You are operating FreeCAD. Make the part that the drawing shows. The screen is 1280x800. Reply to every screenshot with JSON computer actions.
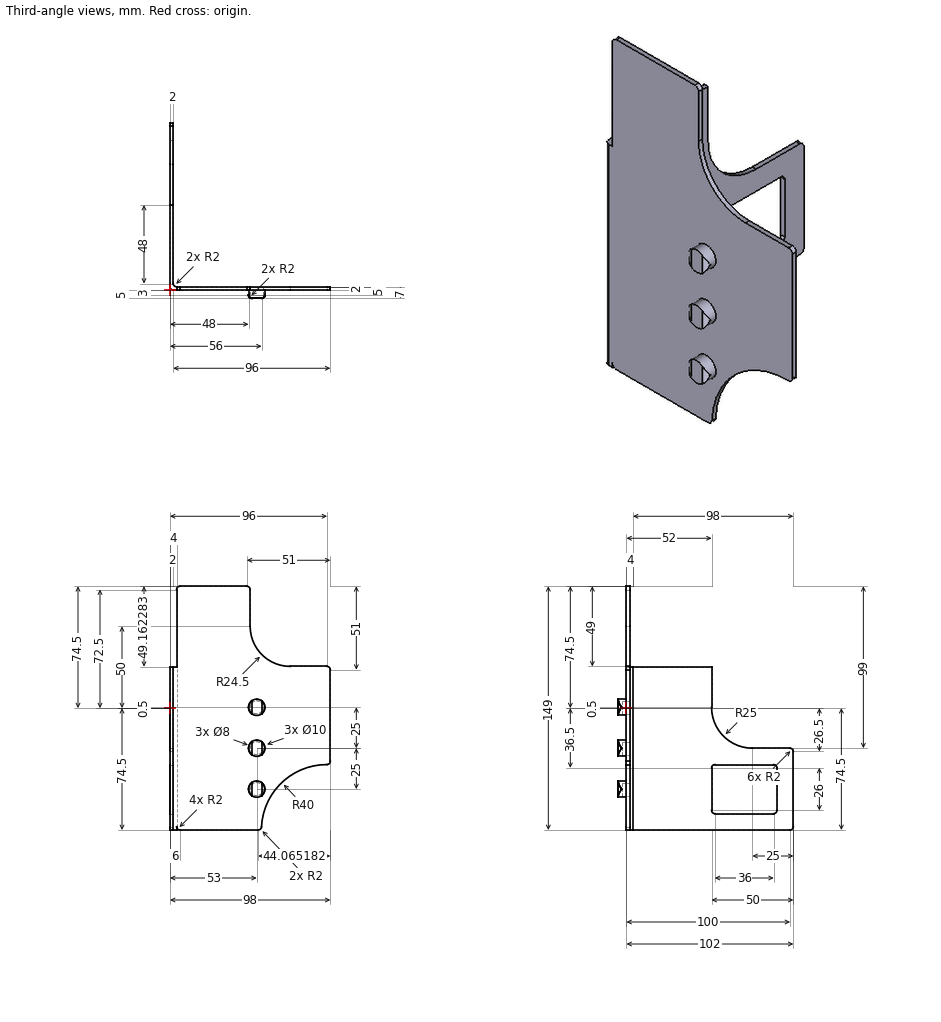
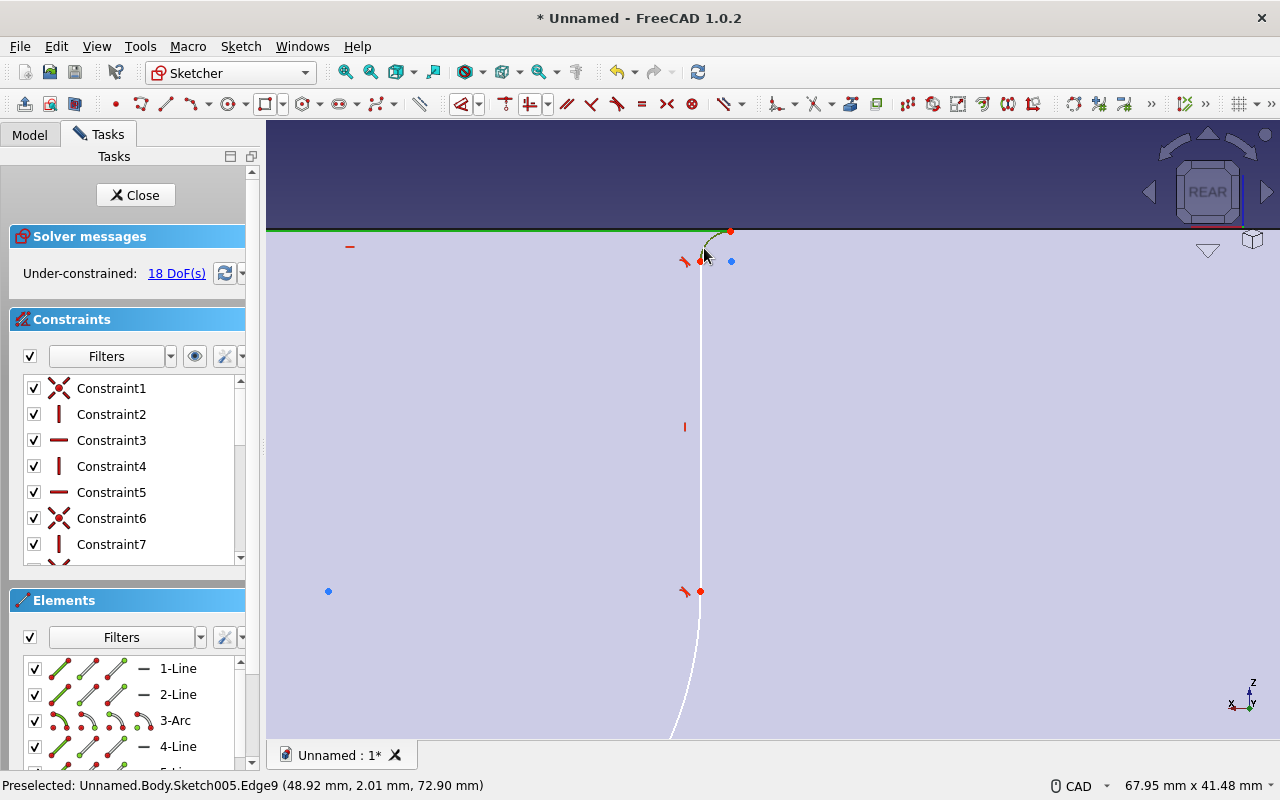
{"action": "key", "text": "t"}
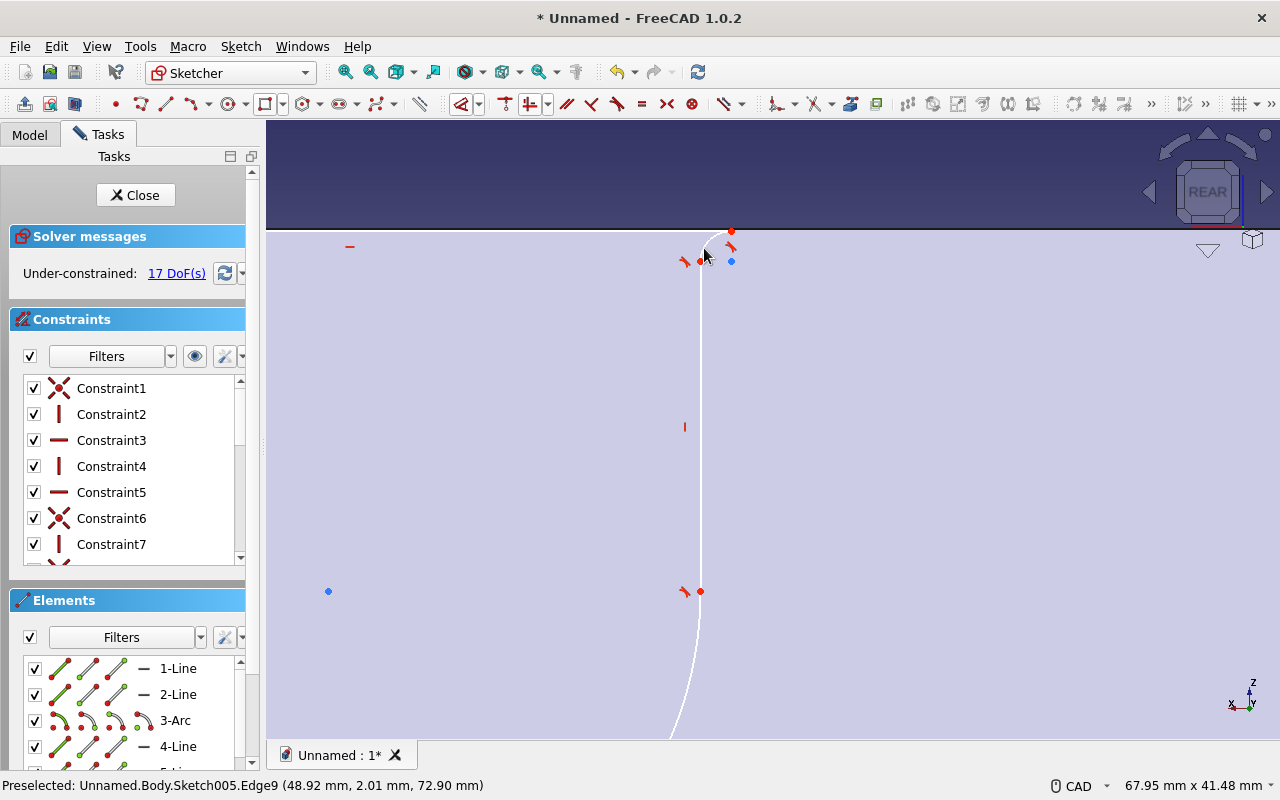
{"action": "scroll", "coordinate": [705, 249], "scroll_direction": "down", "scroll_amount": 9}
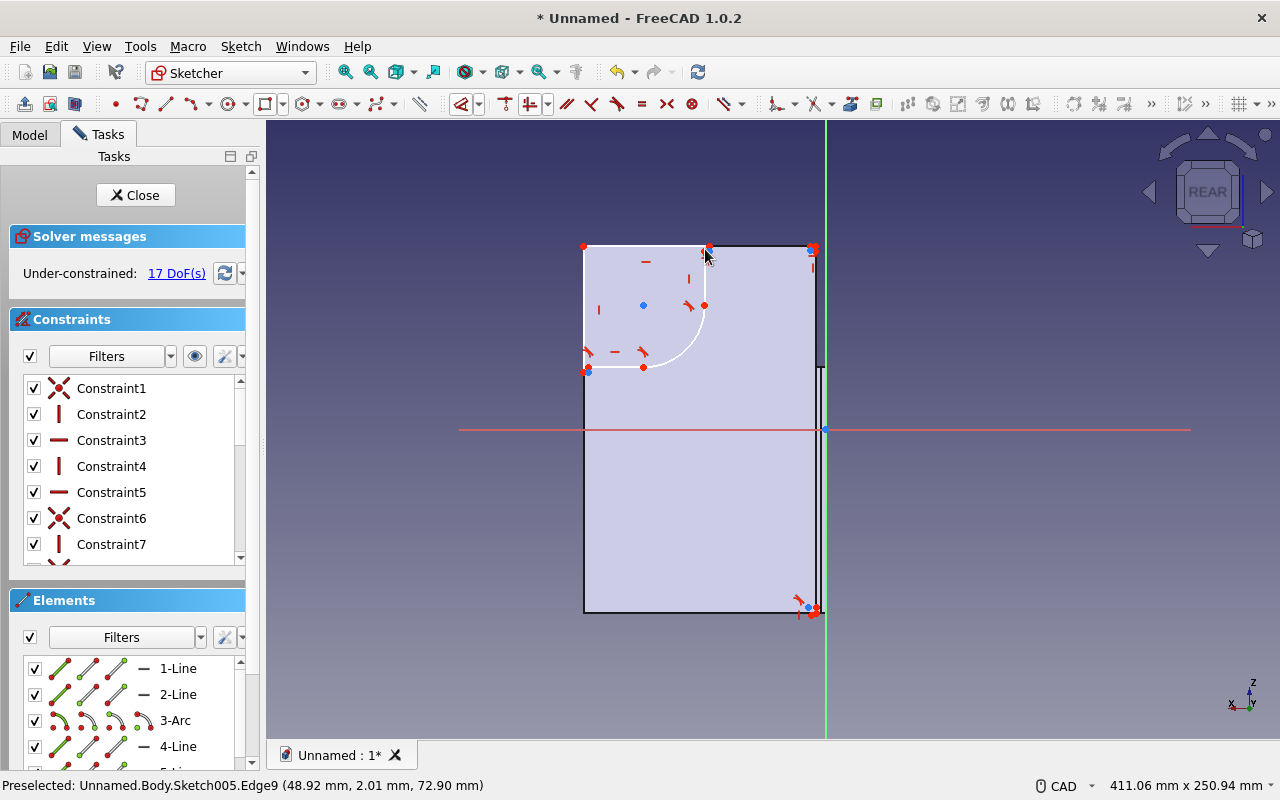
{"action": "left_click", "coordinate": [584, 284]}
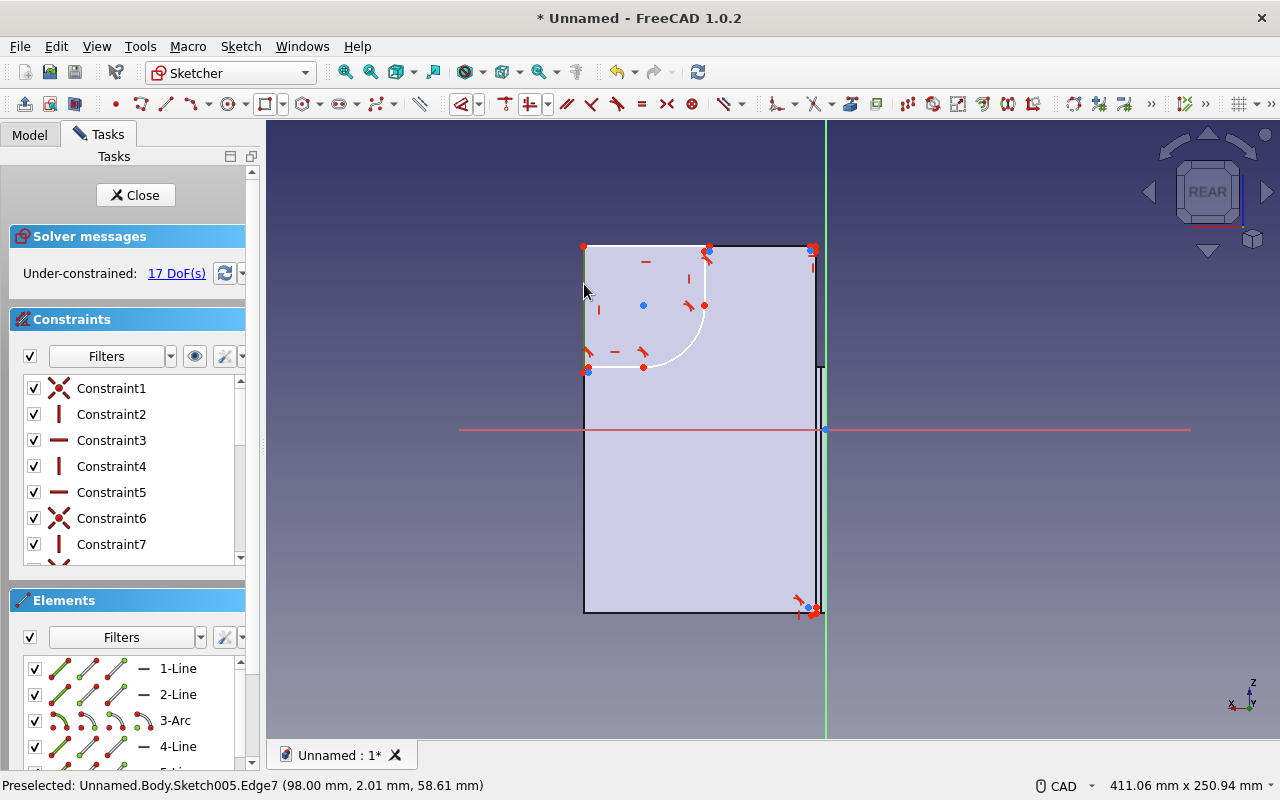
{"action": "scroll", "coordinate": [586, 368], "scroll_direction": "up", "scroll_amount": 10}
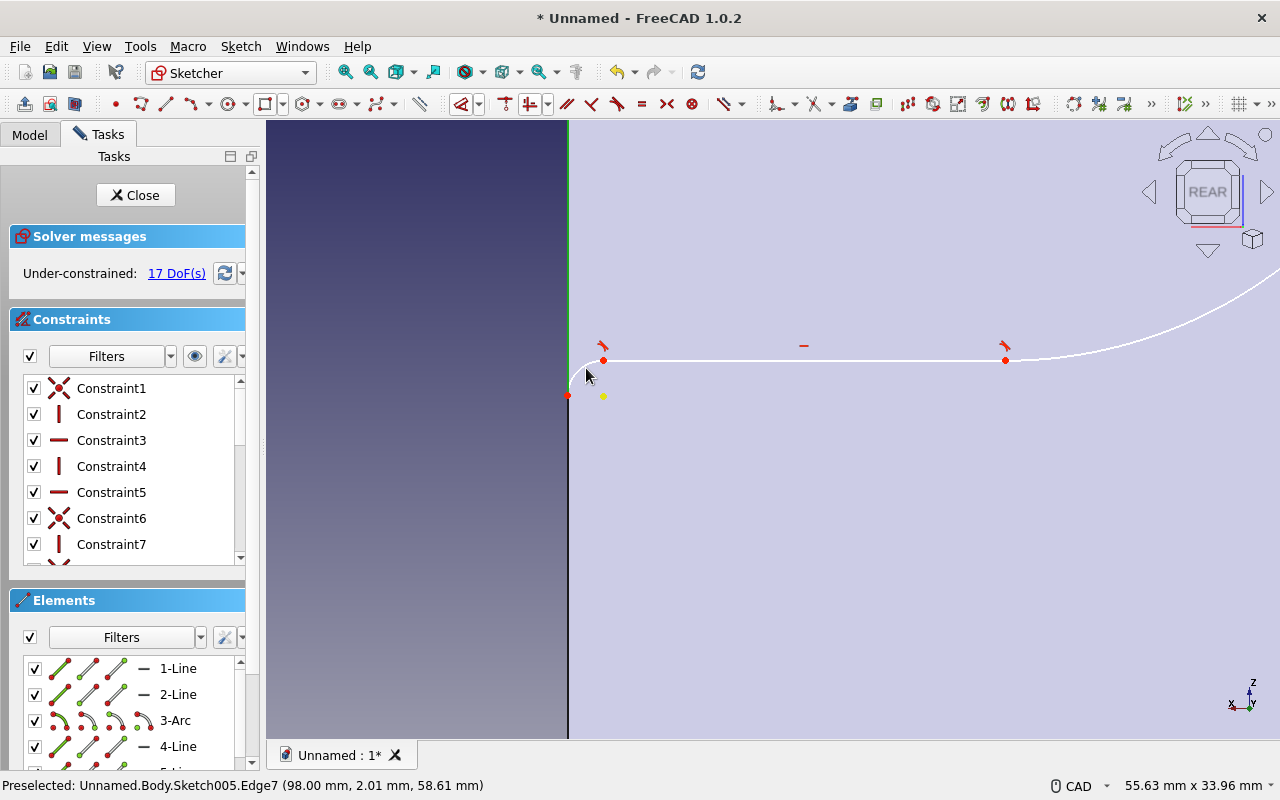
{"action": "left_click", "coordinate": [587, 364]}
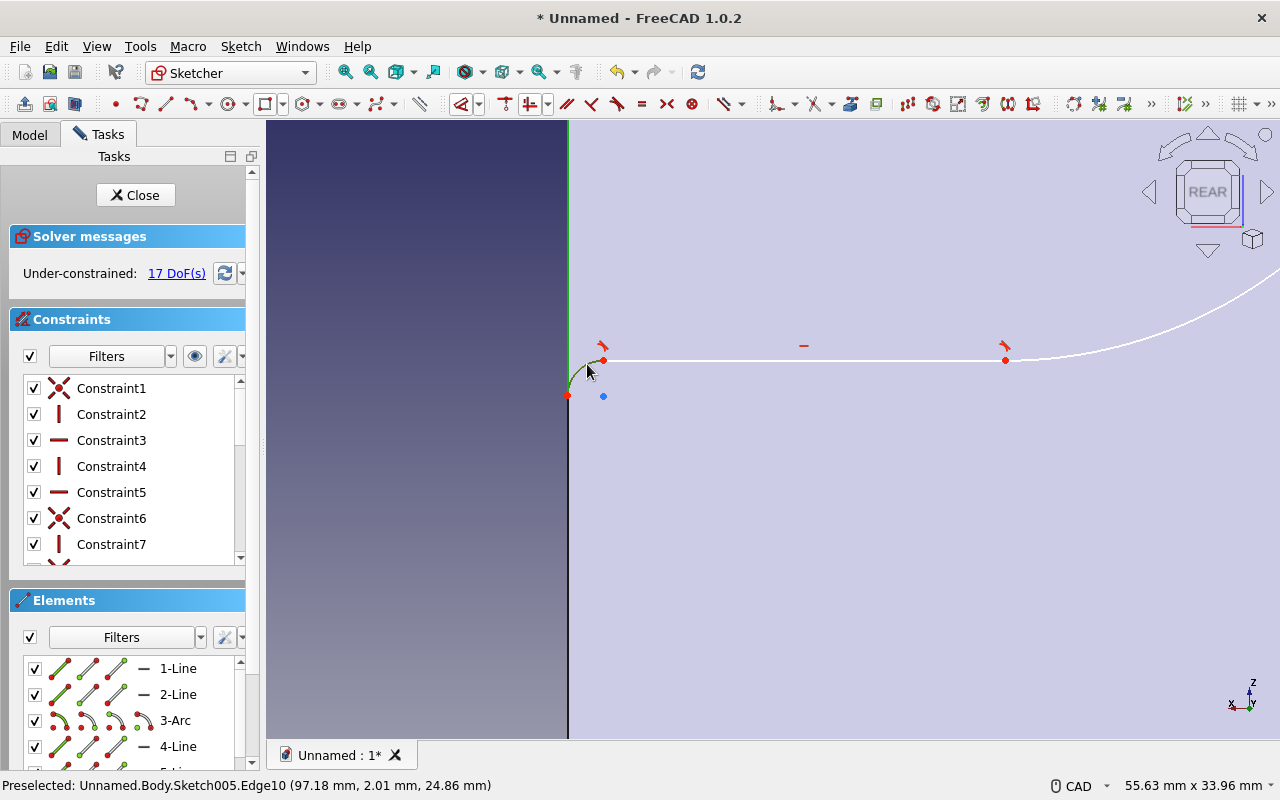
{"action": "left_click", "coordinate": [617, 104]}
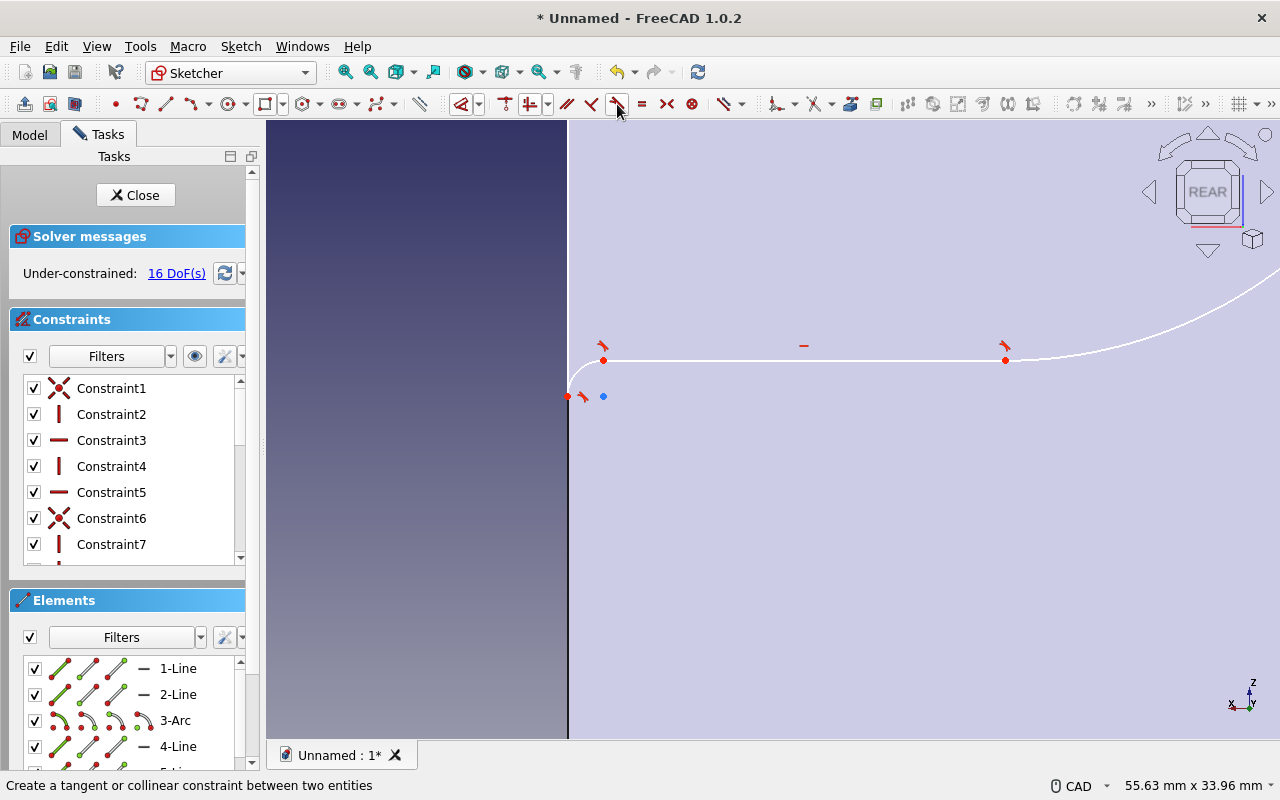
{"action": "scroll", "coordinate": [586, 368], "scroll_direction": "down", "scroll_amount": 10}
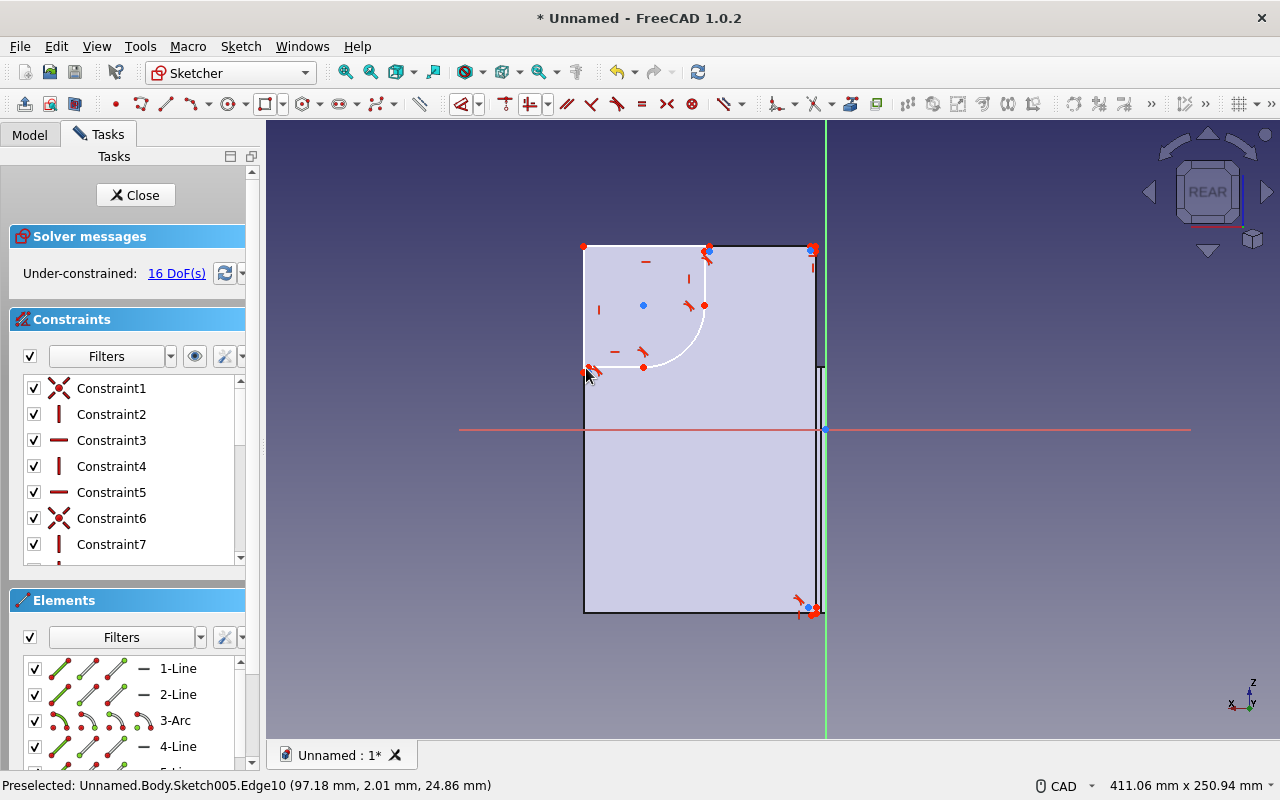
{"action": "scroll", "coordinate": [816, 247], "scroll_direction": "up", "scroll_amount": 13}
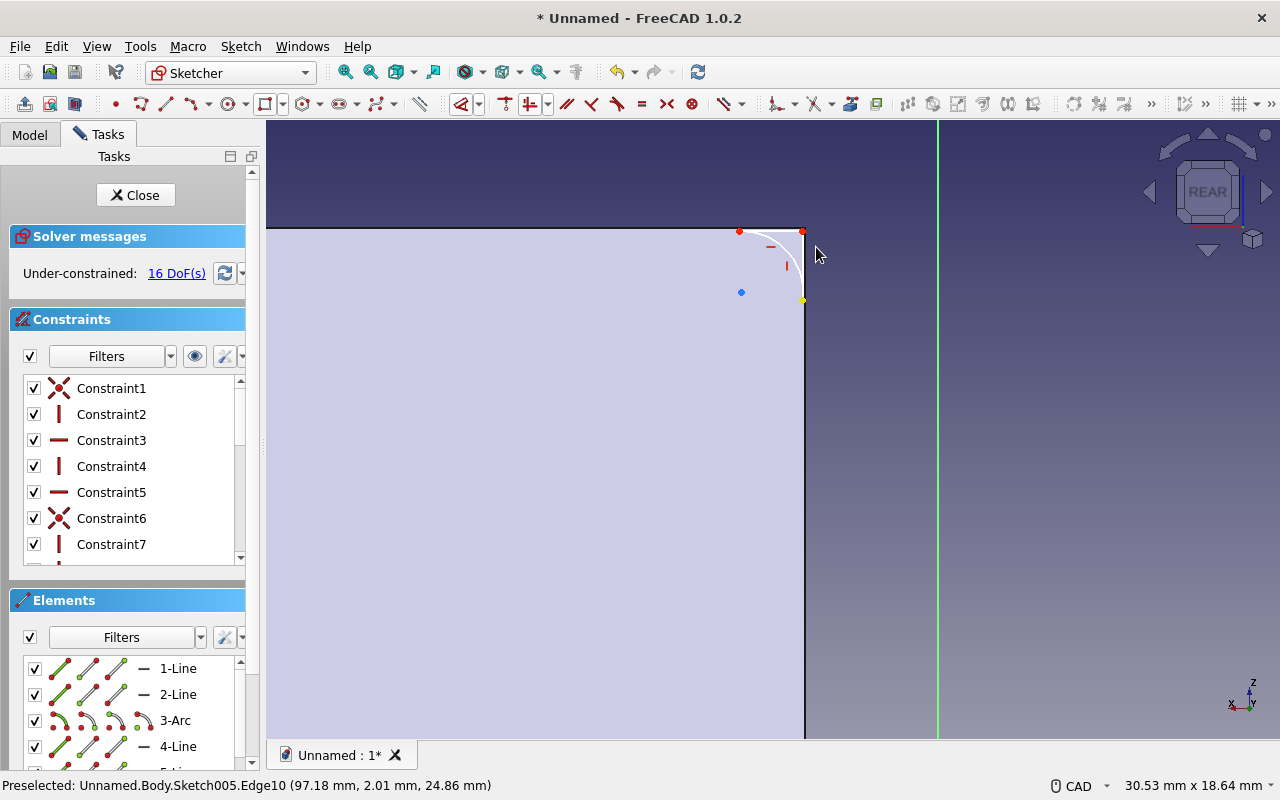
{"action": "left_click", "coordinate": [803, 245]}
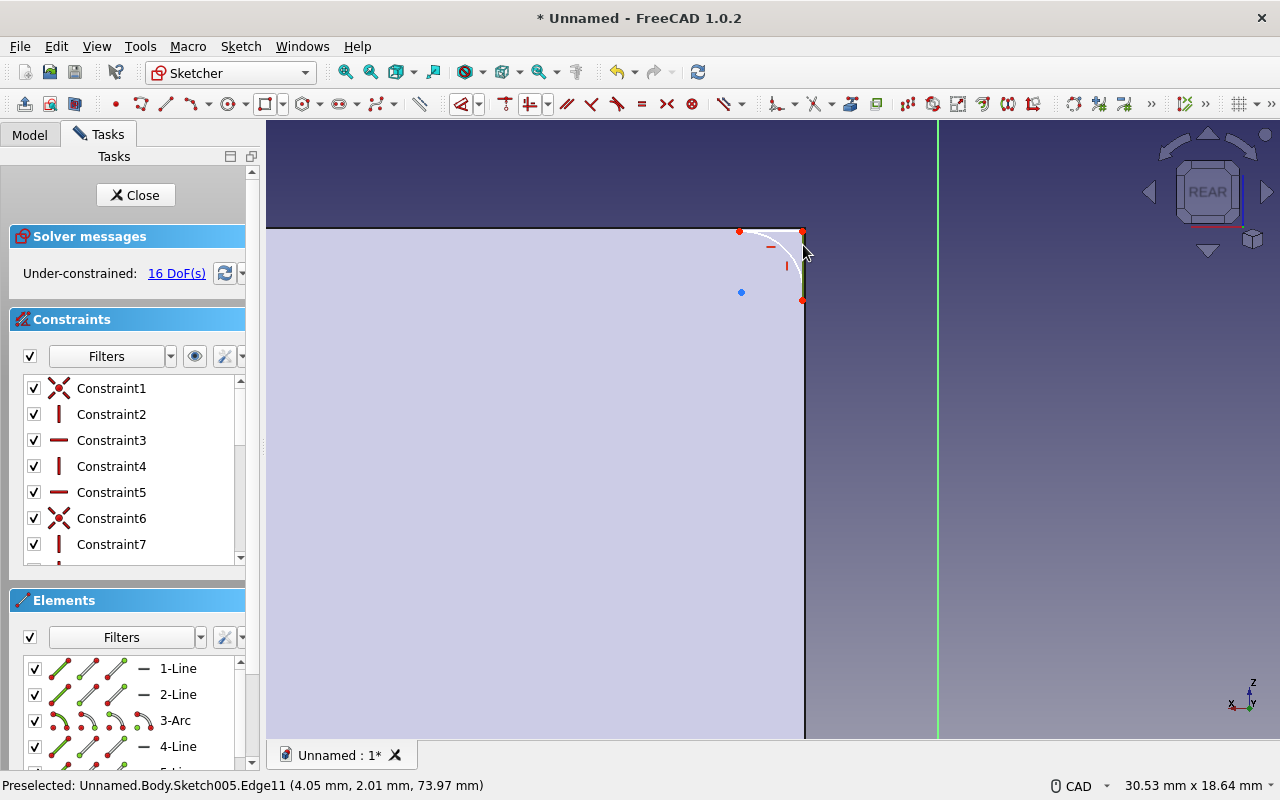
{"action": "left_click", "coordinate": [787, 251]}